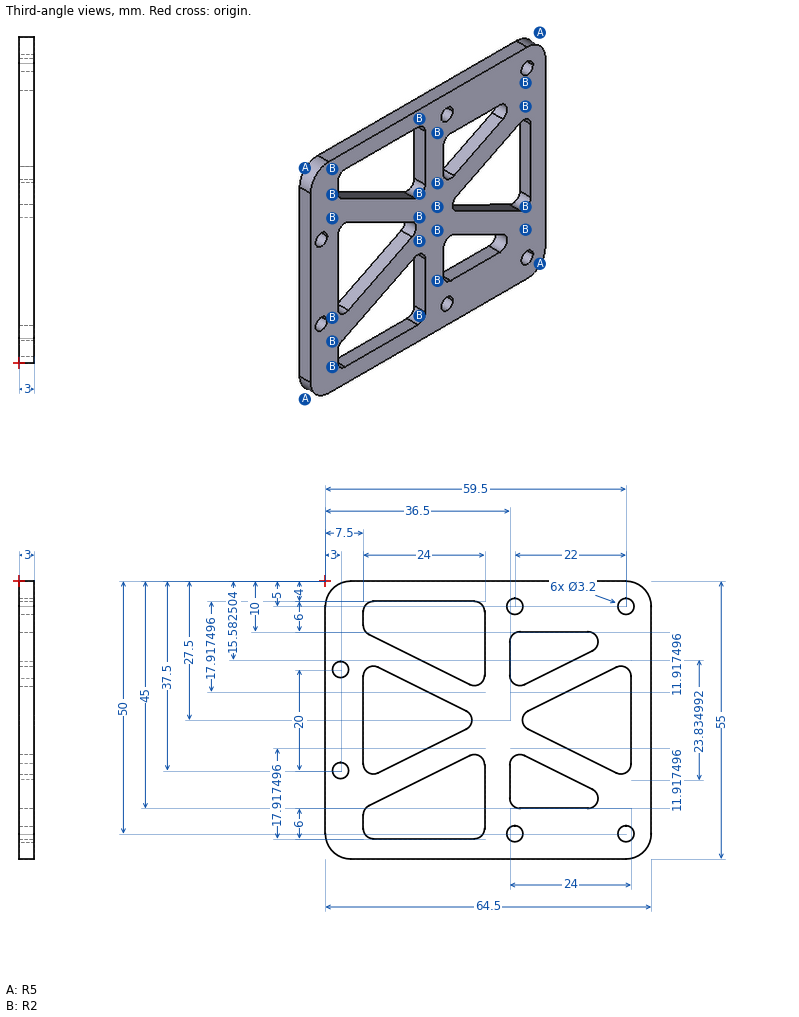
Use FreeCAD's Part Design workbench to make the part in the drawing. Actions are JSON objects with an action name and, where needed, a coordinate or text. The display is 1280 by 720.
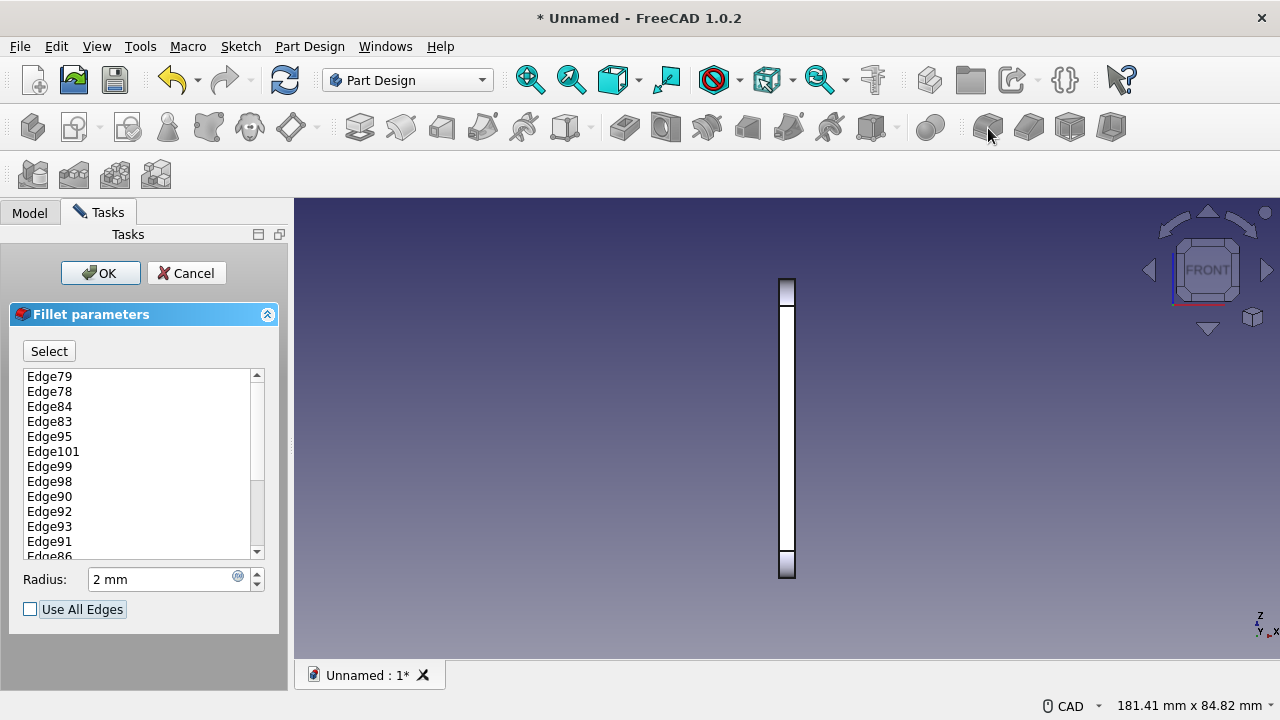
{"action": "left_click", "coordinate": [101, 273]}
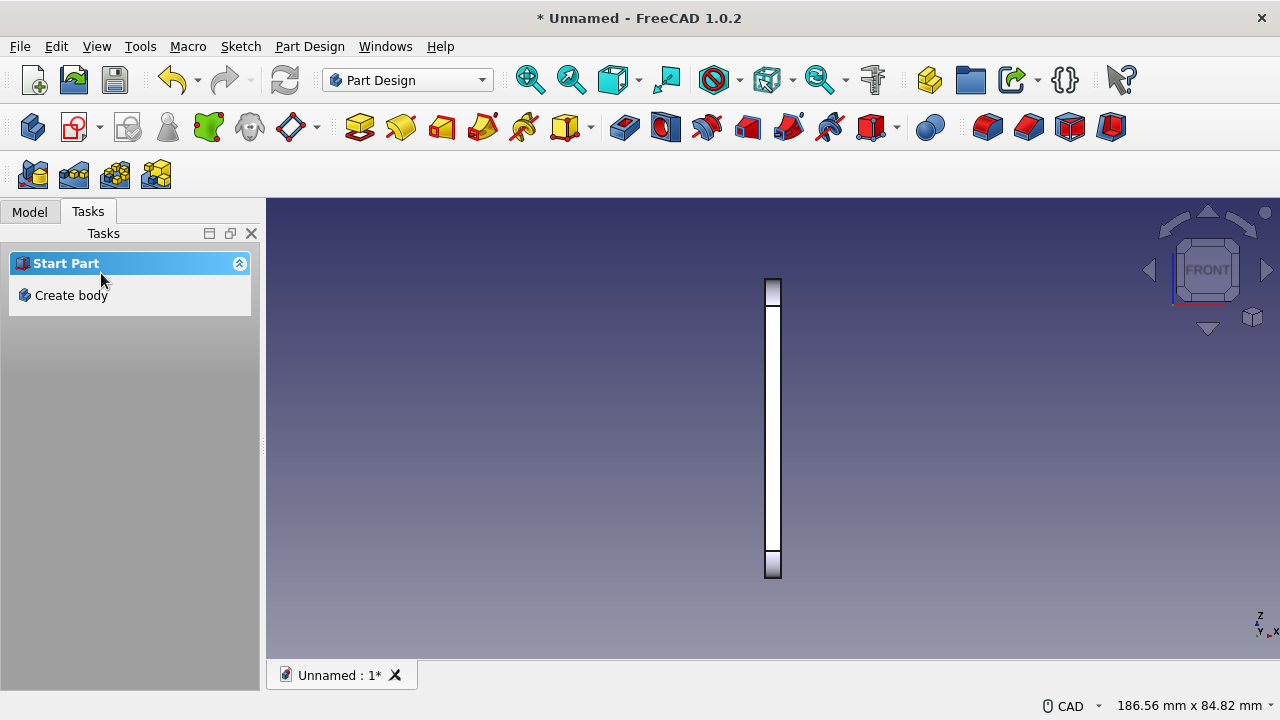
{"action": "key", "text": "0"}